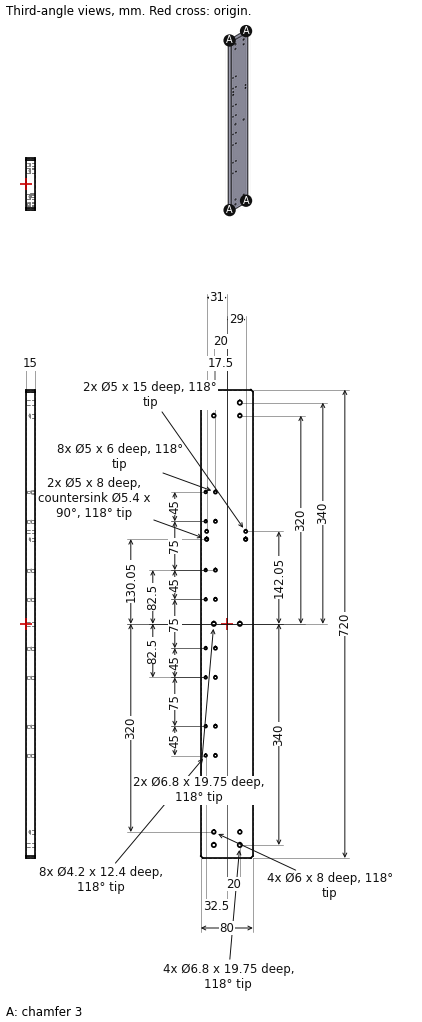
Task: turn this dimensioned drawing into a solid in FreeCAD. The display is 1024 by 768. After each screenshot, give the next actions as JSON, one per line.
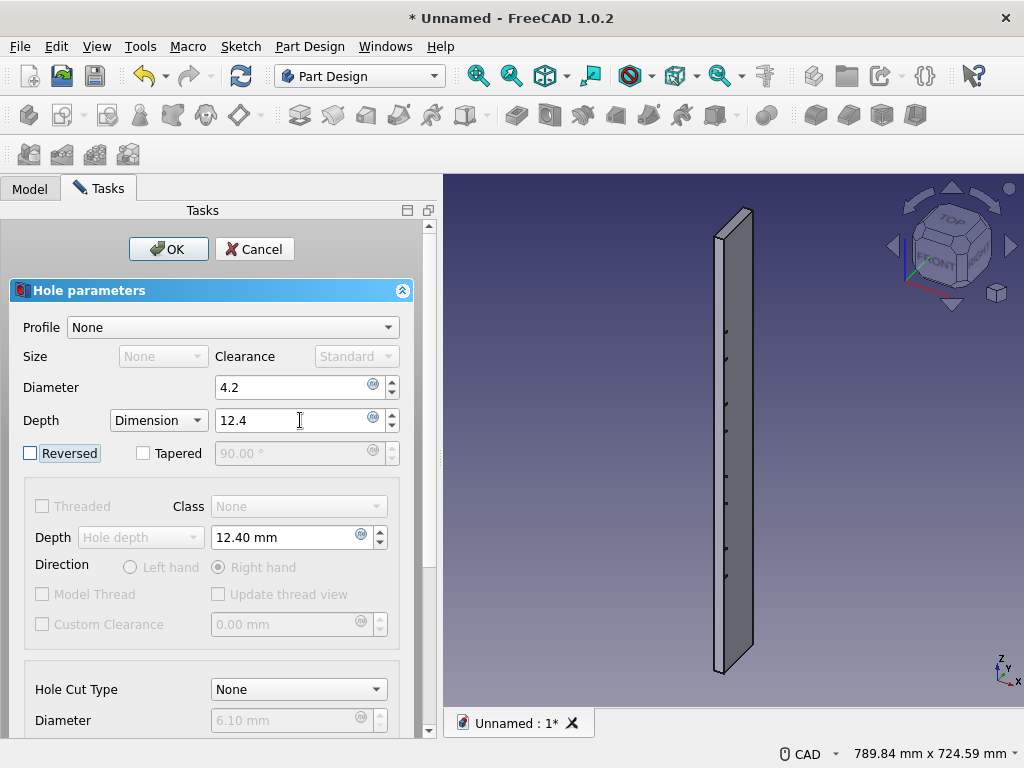
{"action": "left_click", "coordinate": [169, 249]}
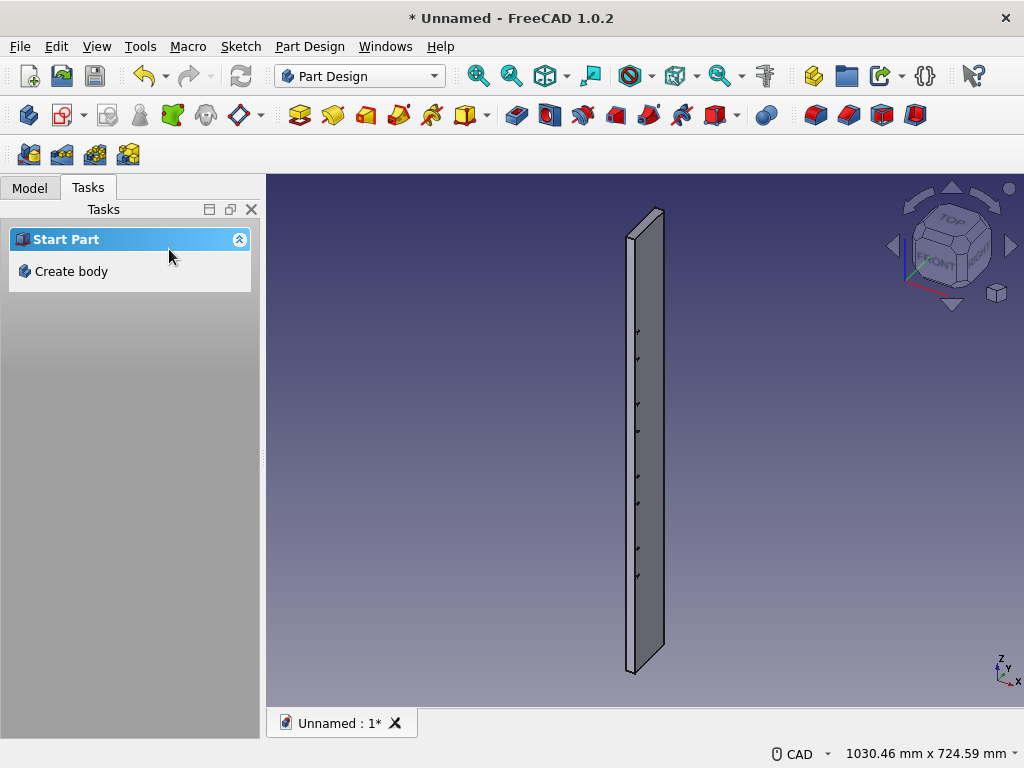
{"action": "left_click", "coordinate": [650, 627]}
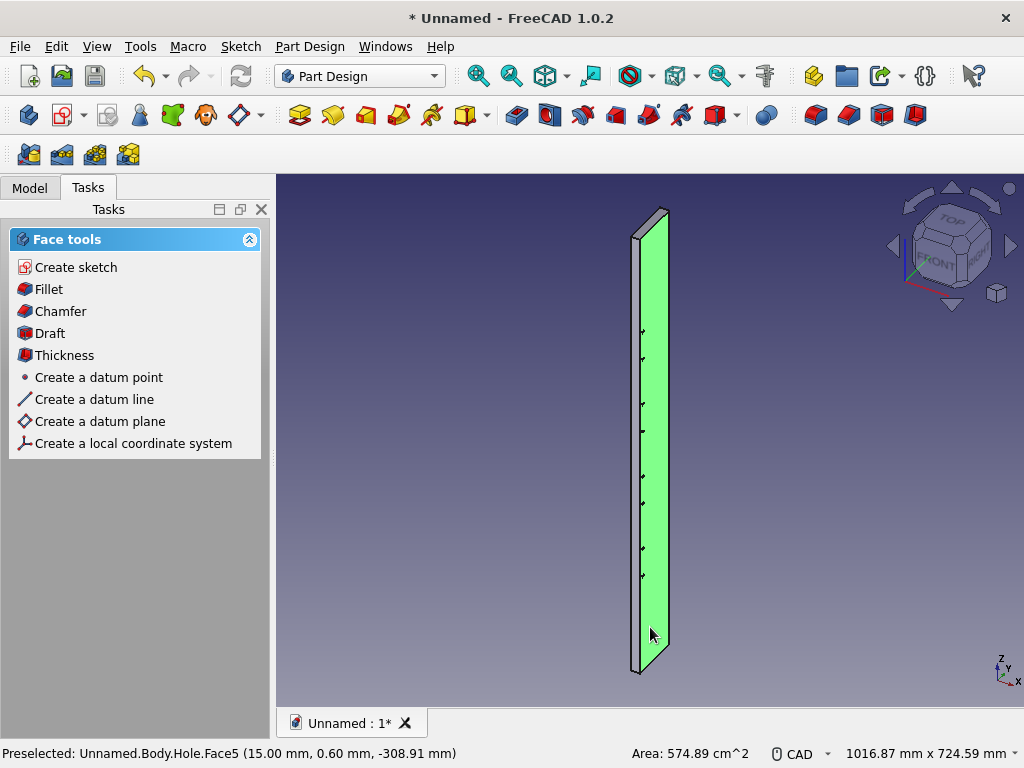
{"action": "left_click", "coordinate": [62, 116]}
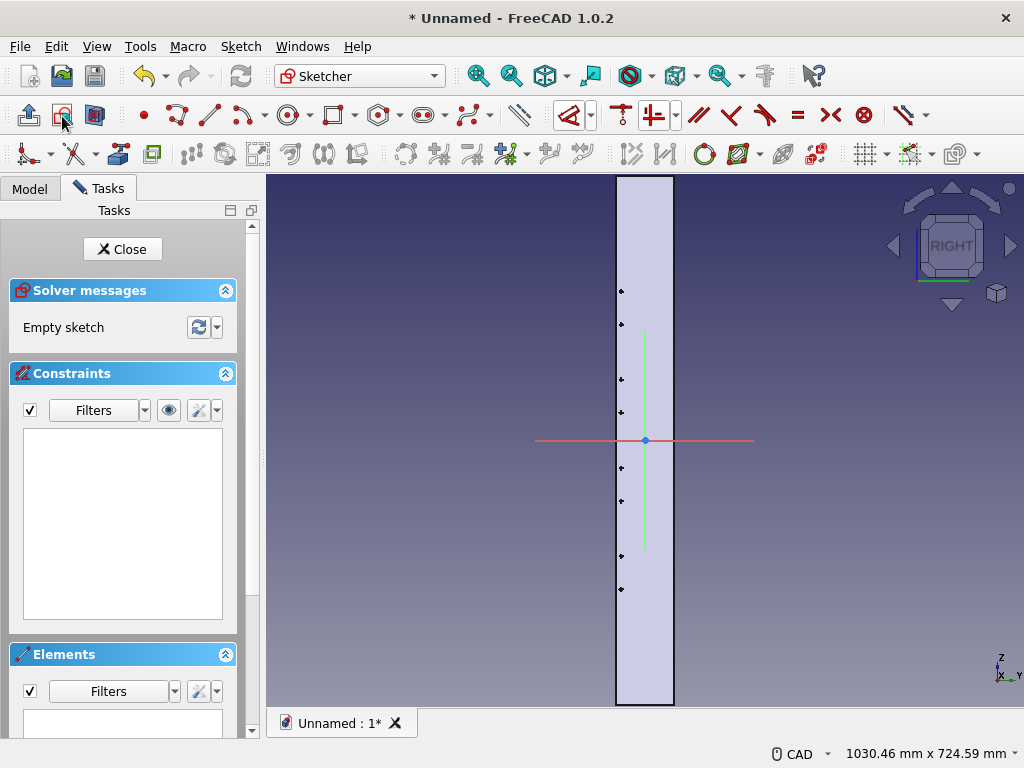
{"action": "left_click", "coordinate": [288, 116]}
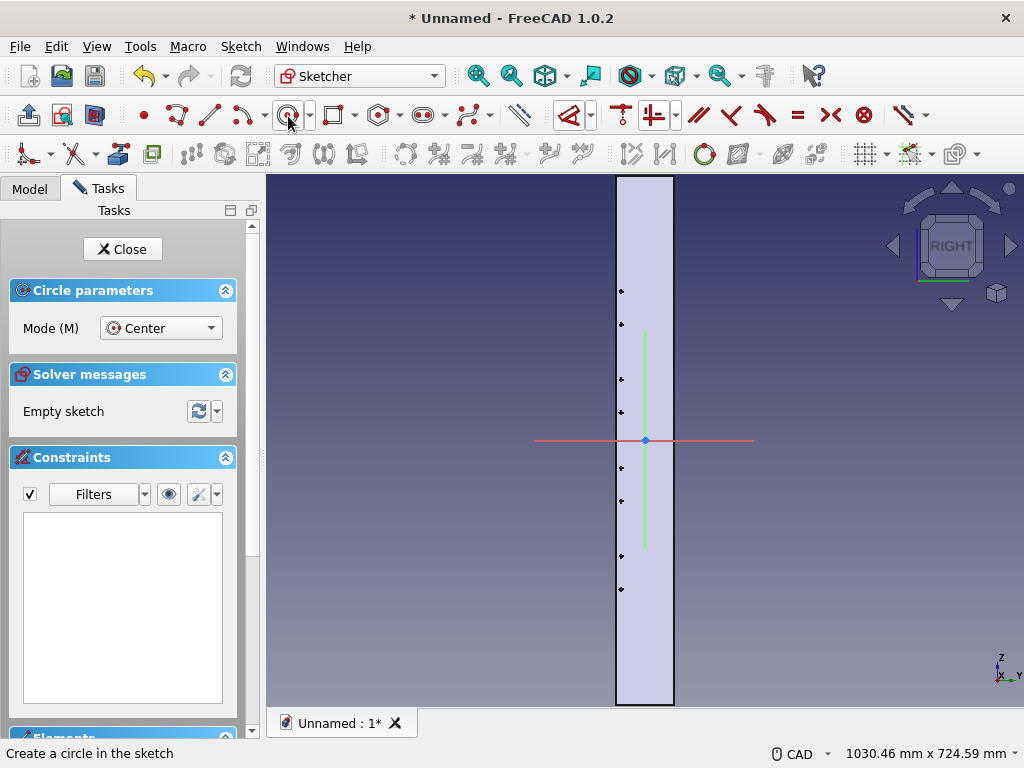
{"action": "scroll", "coordinate": [632, 292], "scroll_direction": "up", "scroll_amount": 13}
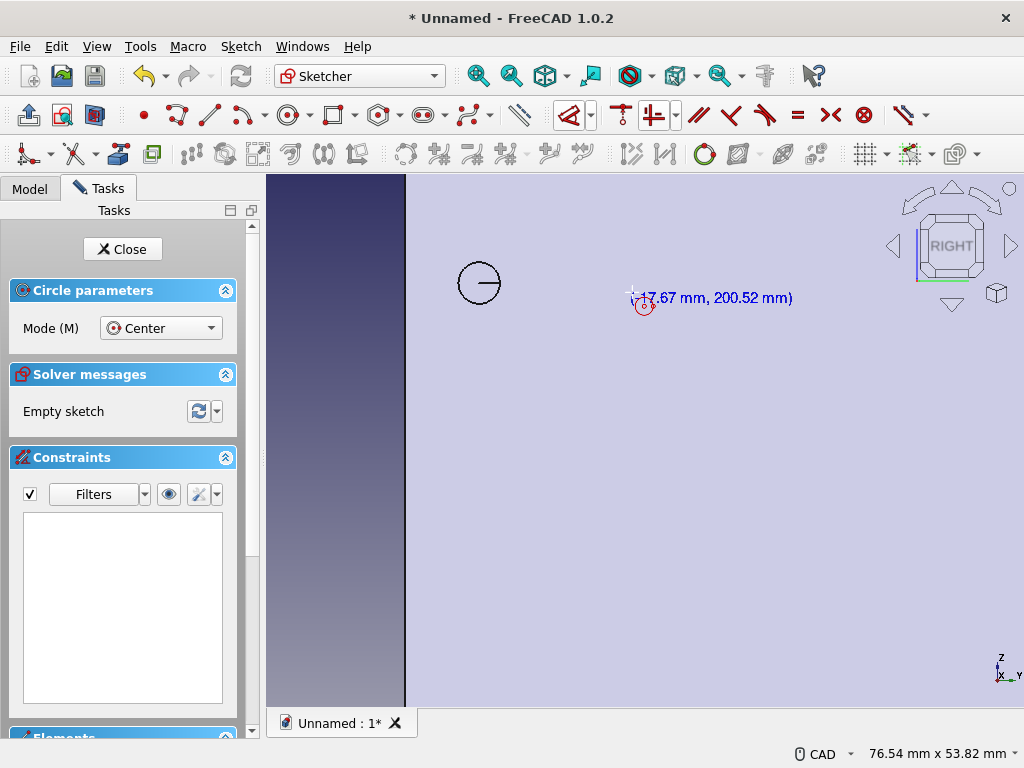
{"action": "scroll", "coordinate": [564, 256], "scroll_direction": "down", "scroll_amount": 12}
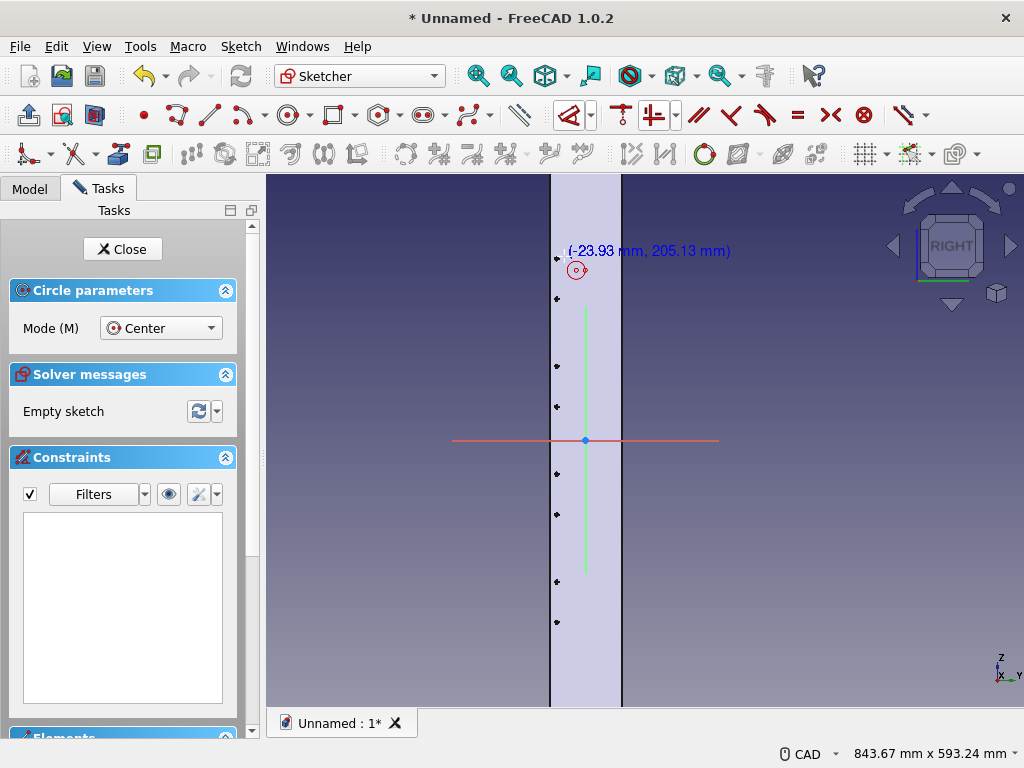
{"action": "left_click", "coordinate": [570, 259]}
{"action": "mouse_move", "coordinate": [572, 257]}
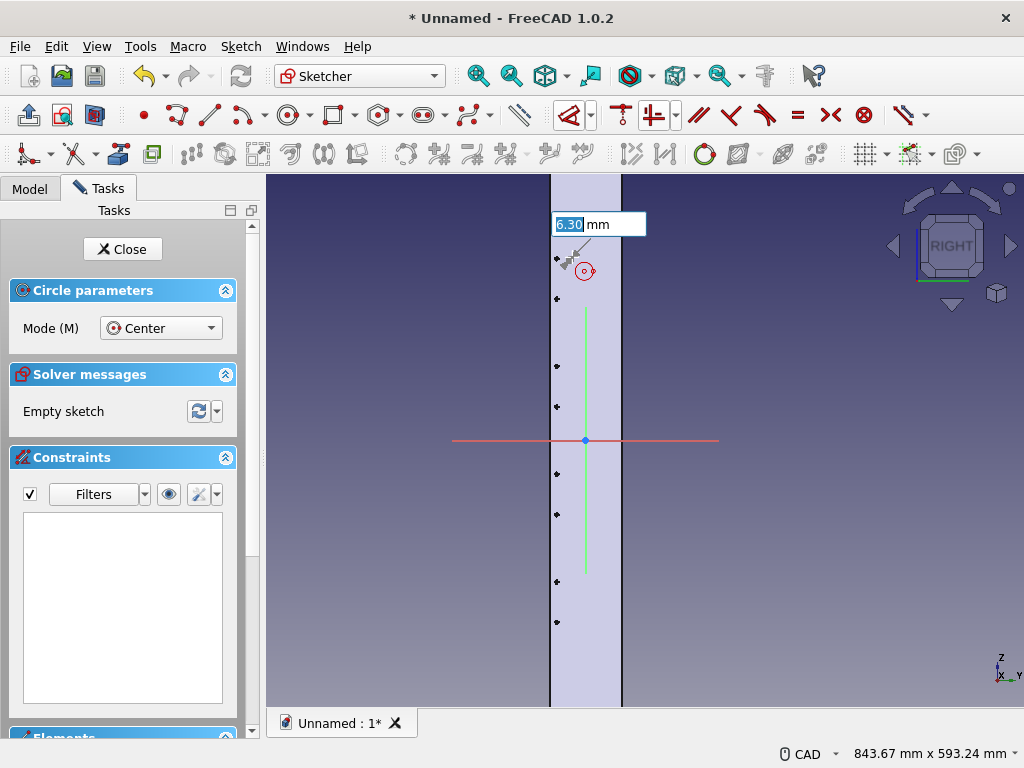
{"action": "type", "text": "5"}
{"action": "key", "text": "Return"}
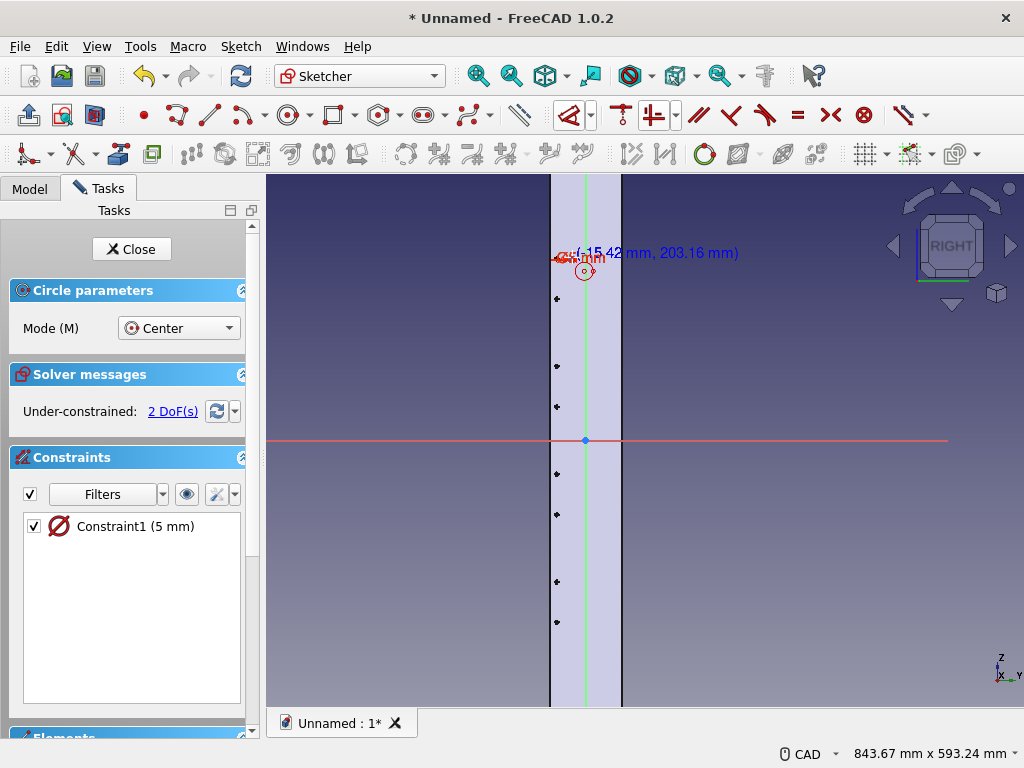
{"action": "scroll", "coordinate": [570, 299], "scroll_direction": "up", "scroll_amount": 12}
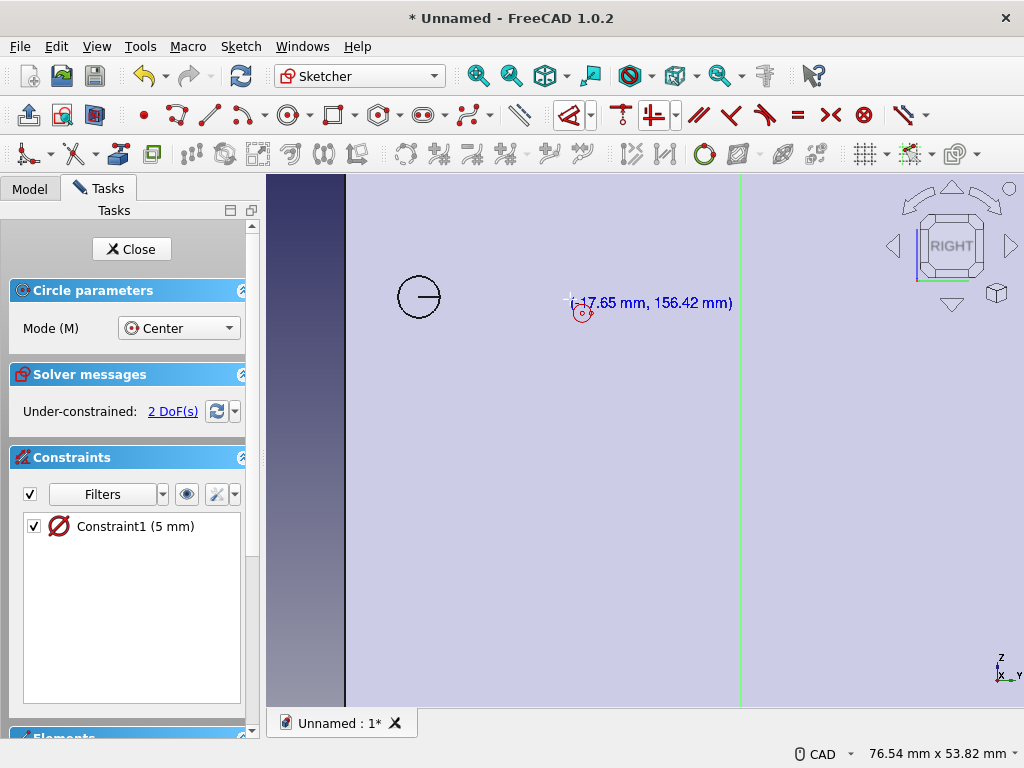
{"action": "scroll", "coordinate": [570, 299], "scroll_direction": "down", "scroll_amount": 12}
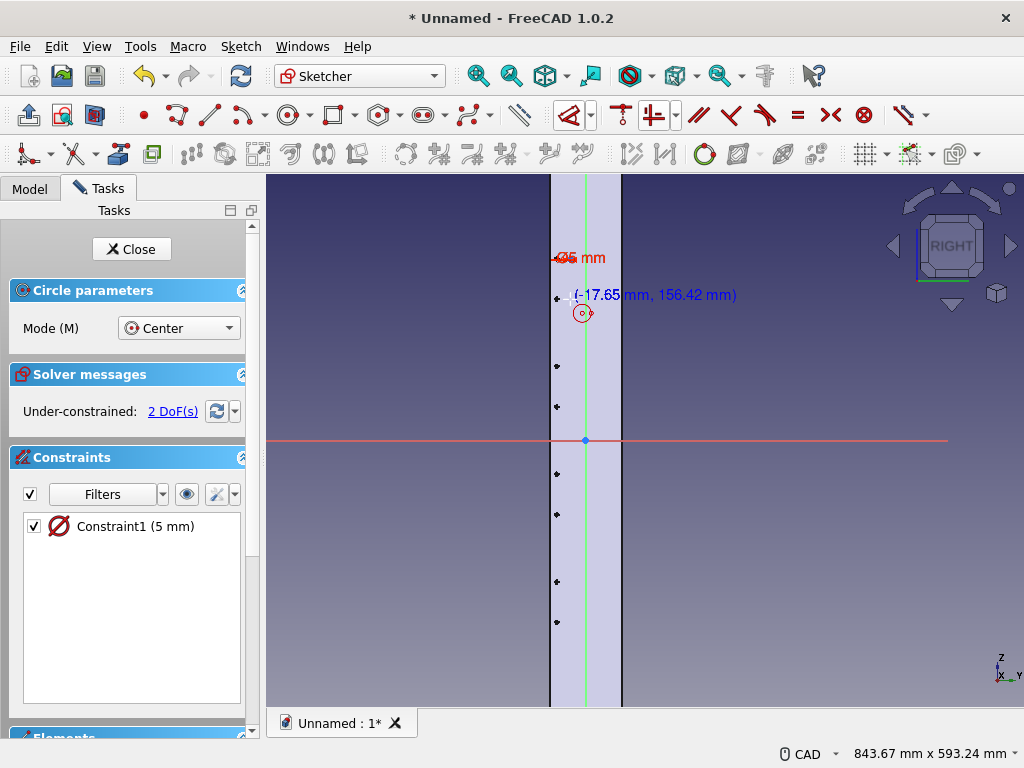
{"action": "left_click", "coordinate": [570, 299]}
{"action": "mouse_move", "coordinate": [572, 297]}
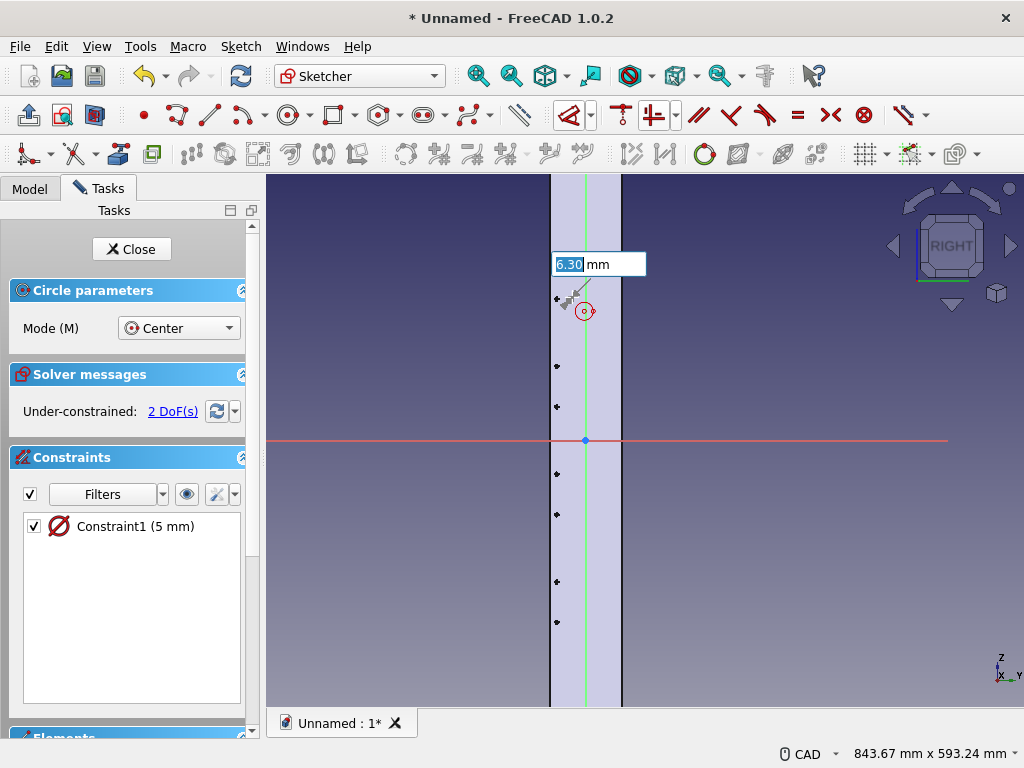
{"action": "type", "text": "5"}
{"action": "key", "text": "Return"}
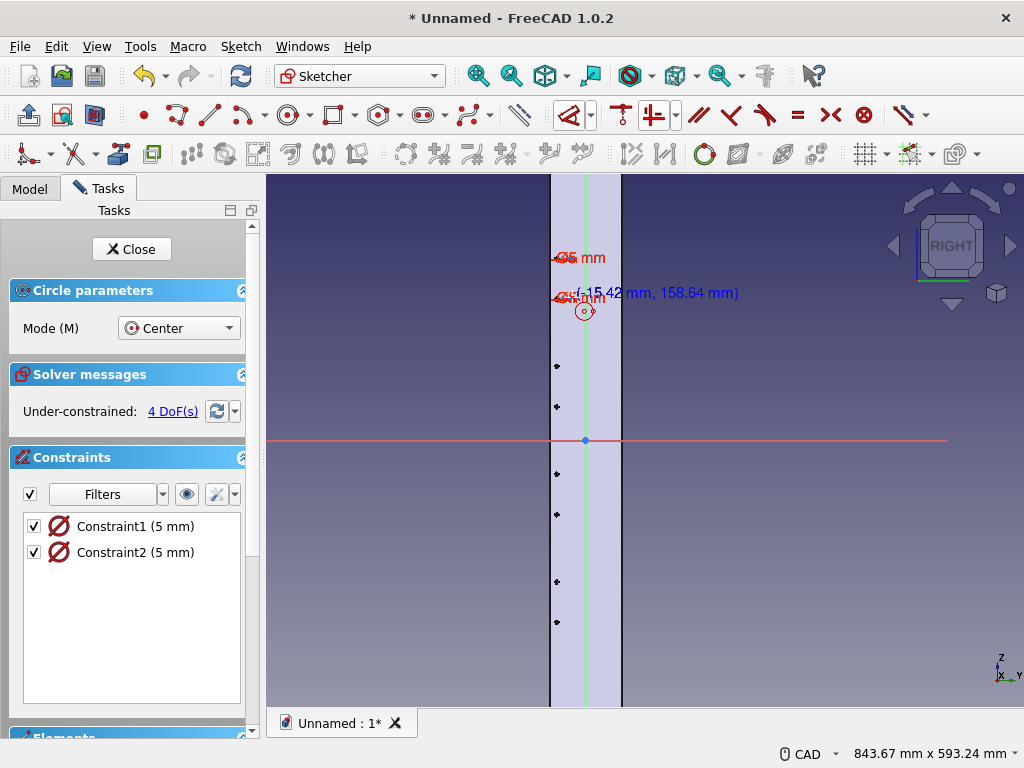
{"action": "scroll", "coordinate": [570, 366], "scroll_direction": "up", "scroll_amount": 12}